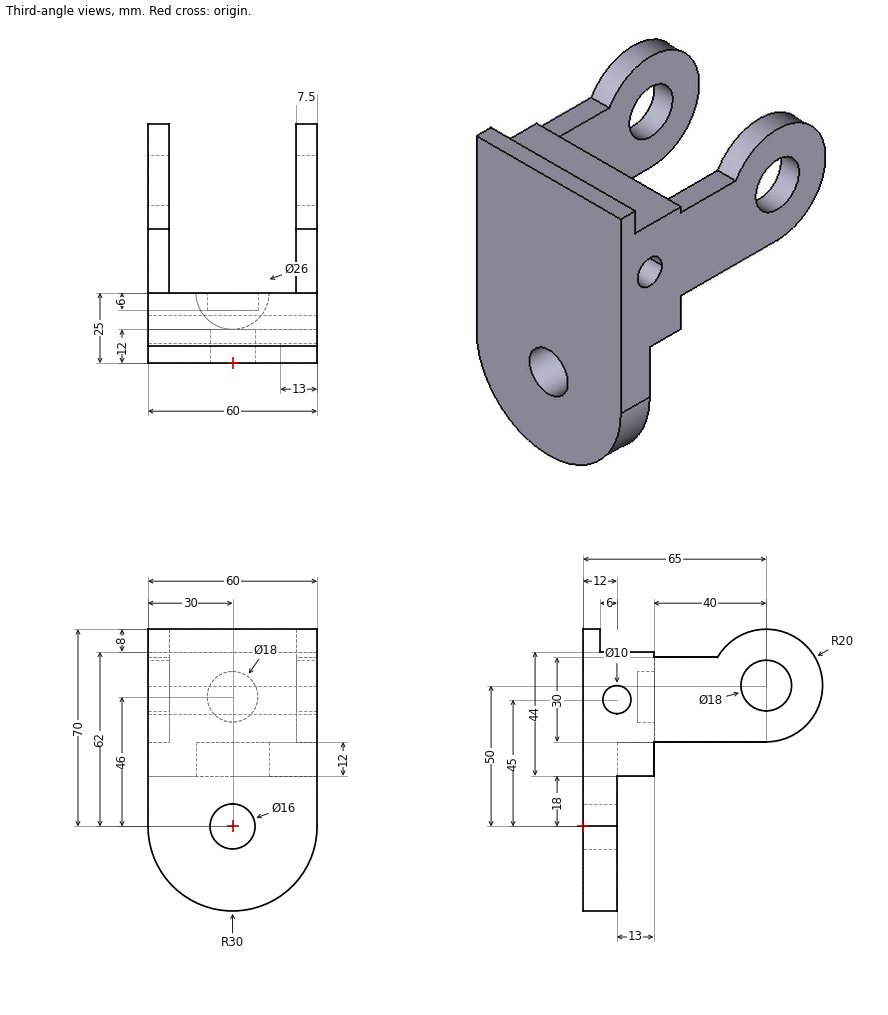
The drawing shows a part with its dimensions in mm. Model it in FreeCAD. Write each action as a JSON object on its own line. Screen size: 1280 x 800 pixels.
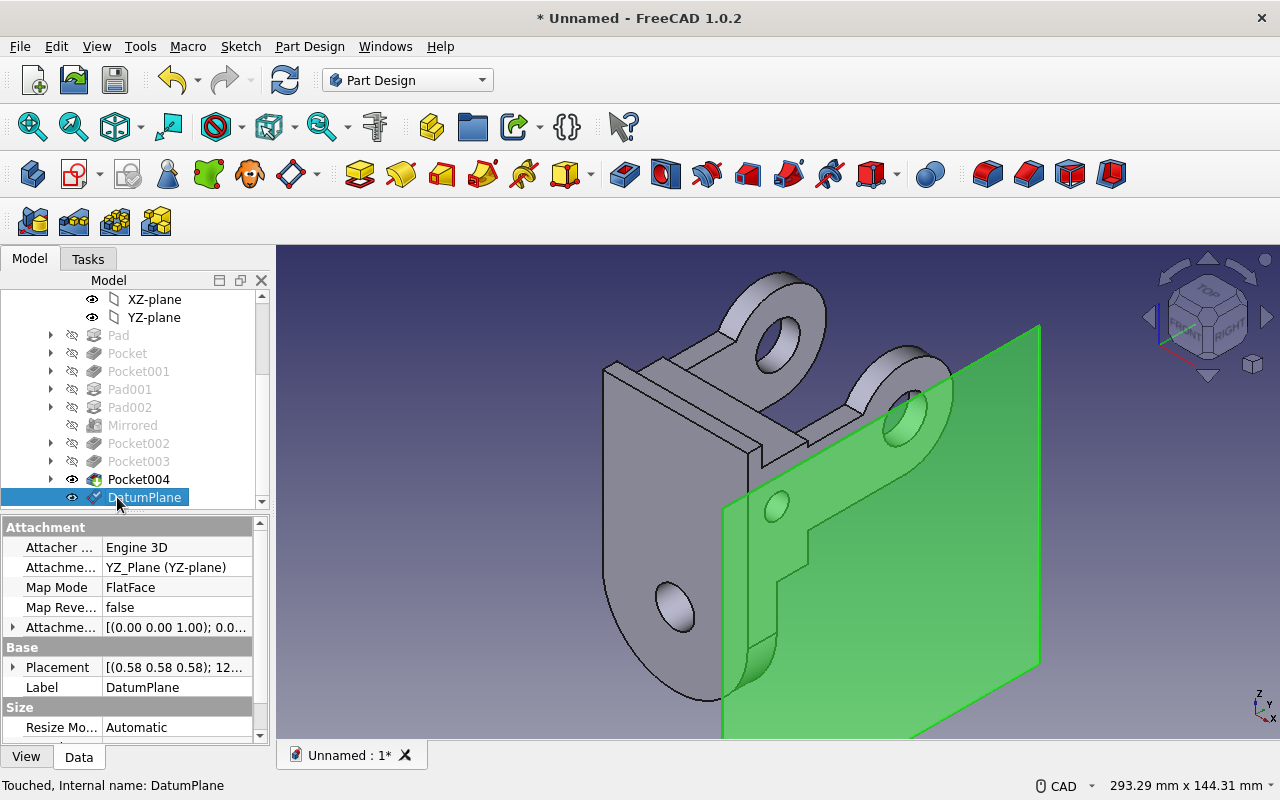
{"action": "left_click", "coordinate": [74, 174]}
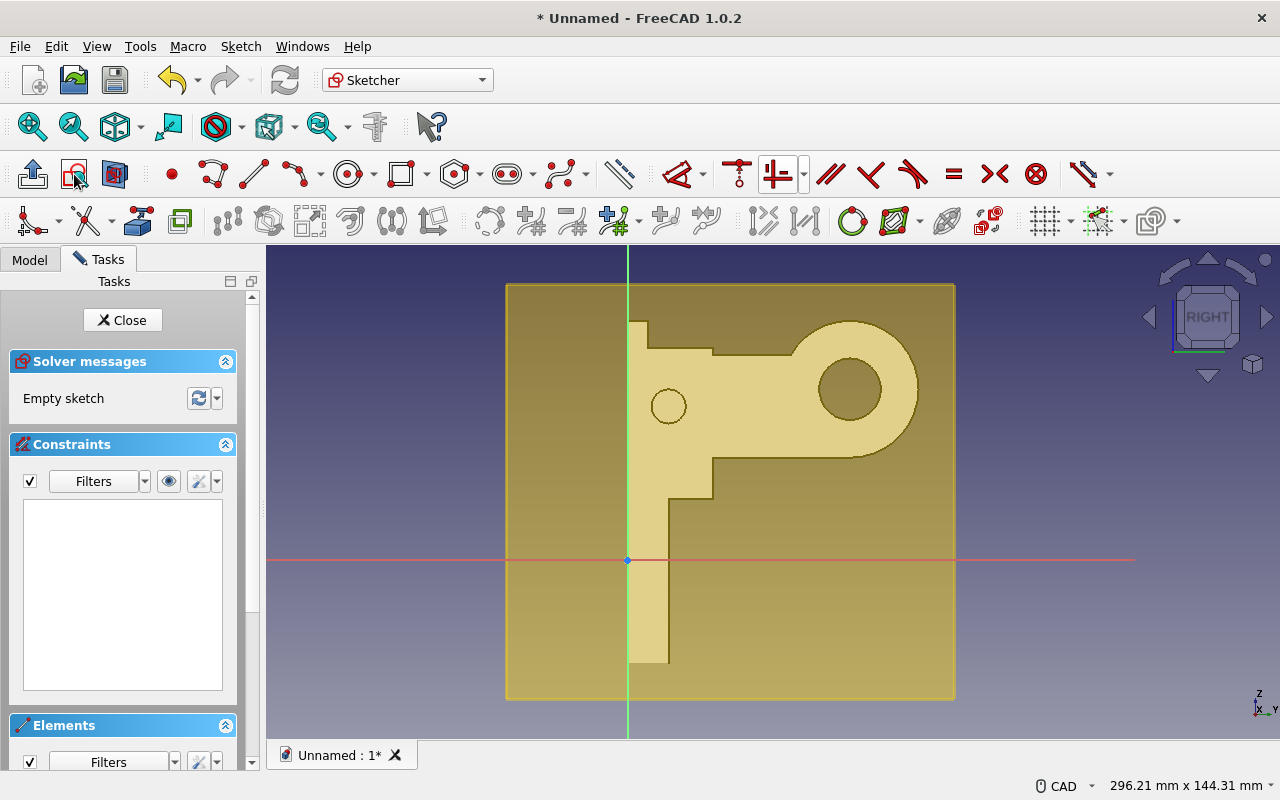
{"action": "scroll", "coordinate": [664, 396], "scroll_direction": "up", "scroll_amount": 11}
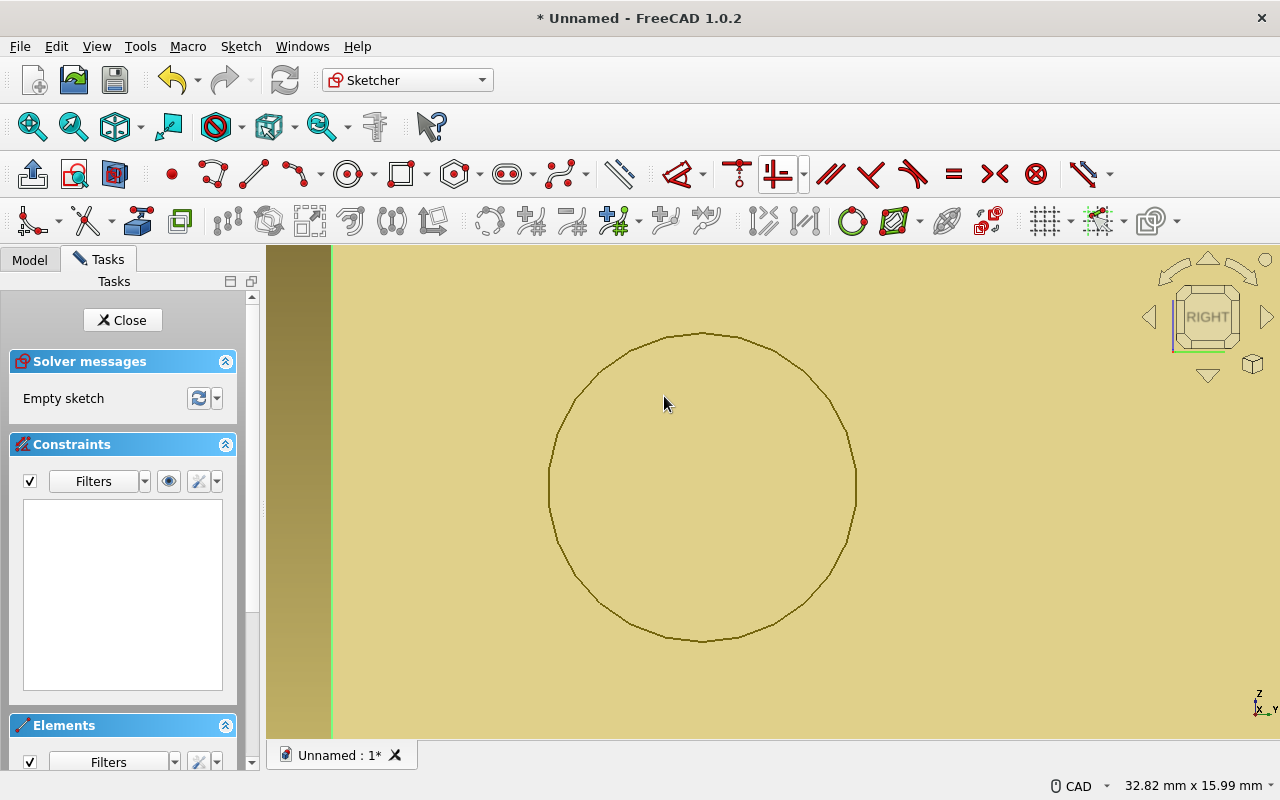
{"action": "left_click", "coordinate": [348, 174]}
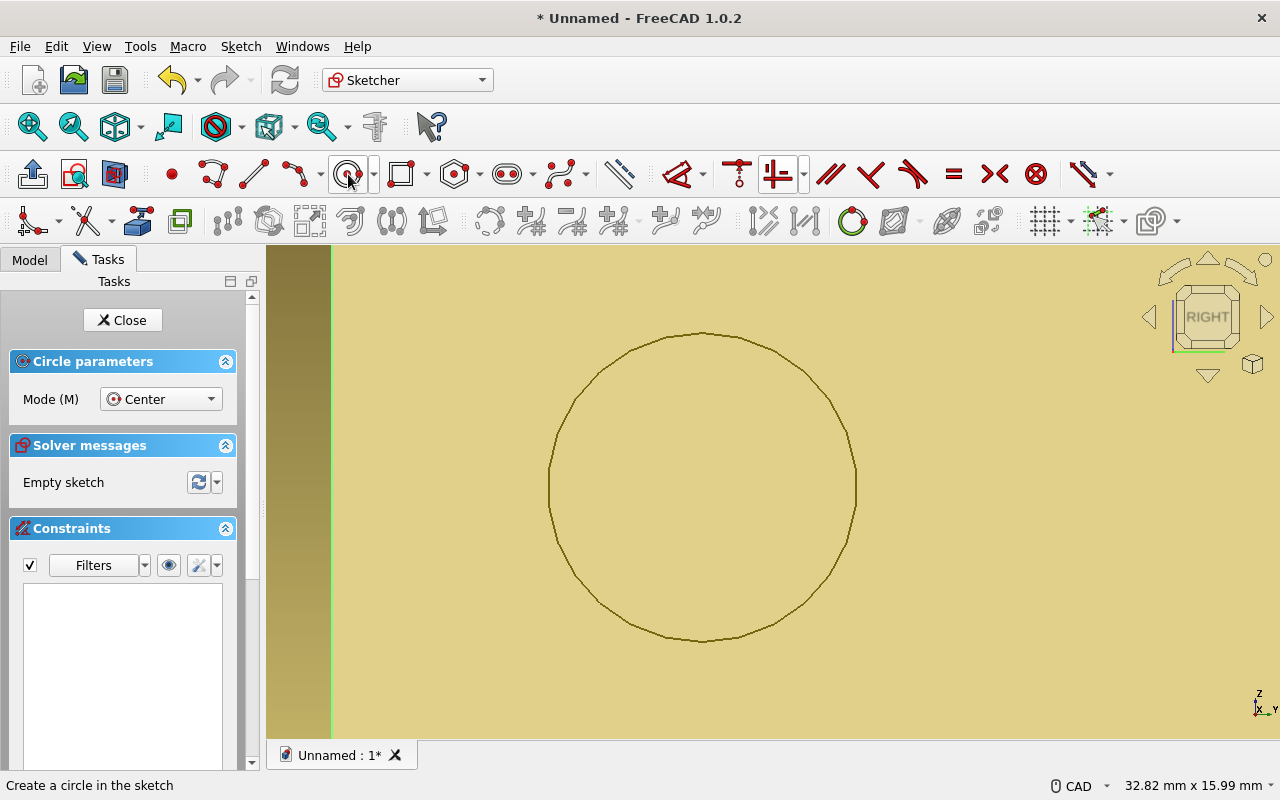
{"action": "left_click", "coordinate": [702, 488]}
{"action": "left_click", "coordinate": [812, 378]}
{"action": "key", "text": "Escape"}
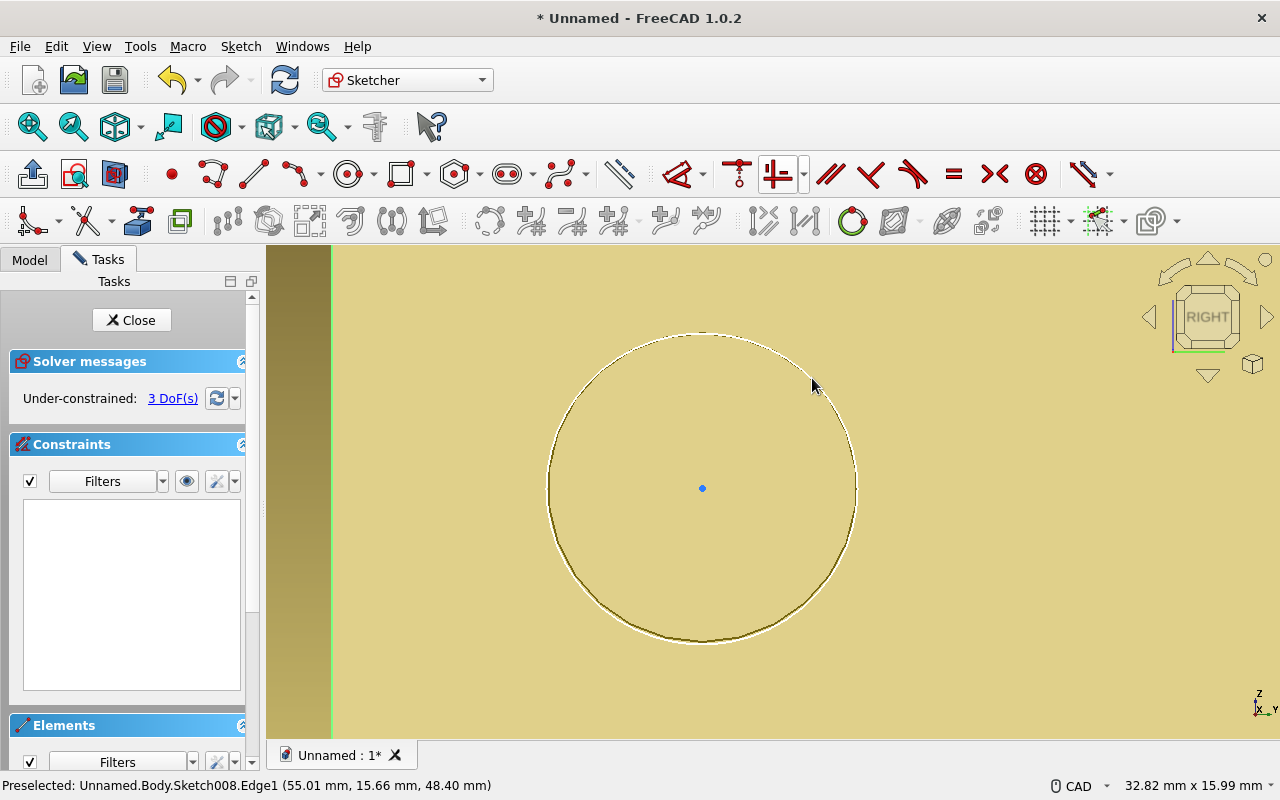
{"action": "key", "text": "d"}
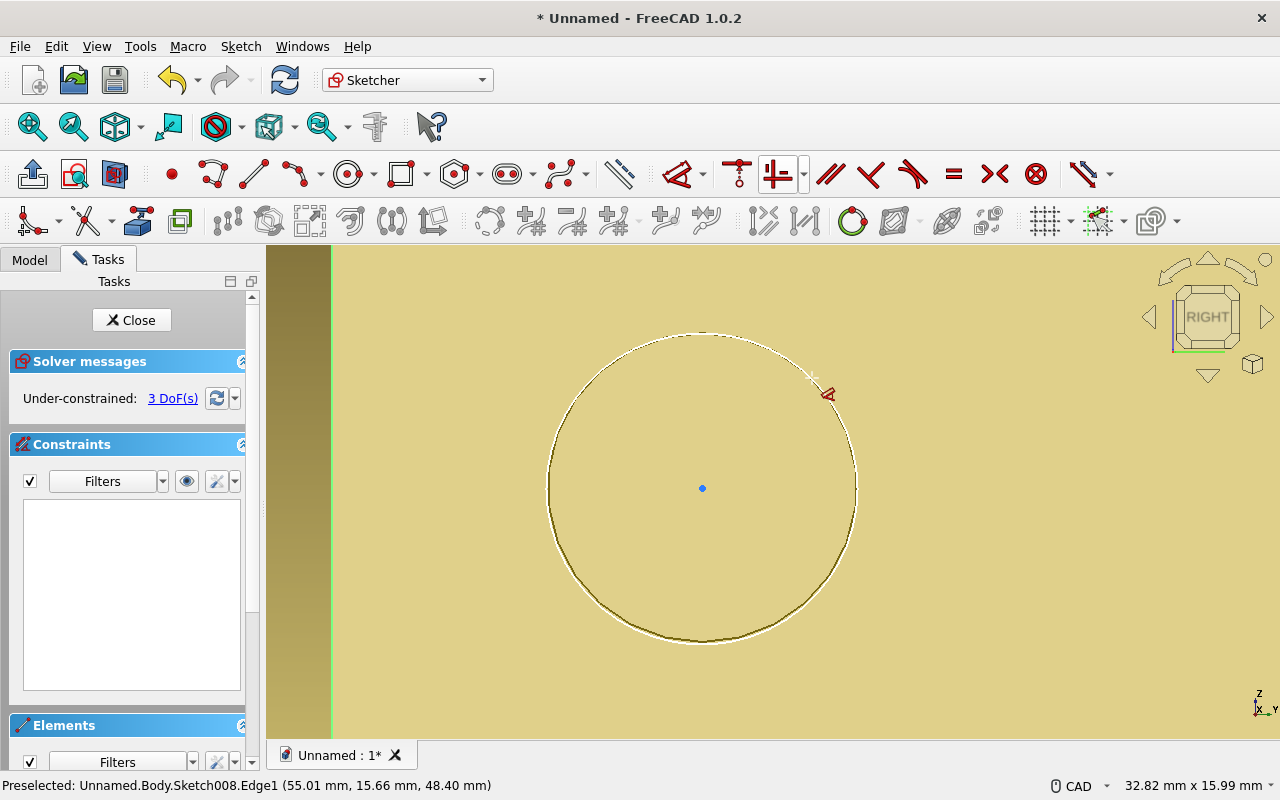
{"action": "left_click", "coordinate": [812, 379]}
{"action": "left_click", "coordinate": [835, 356]}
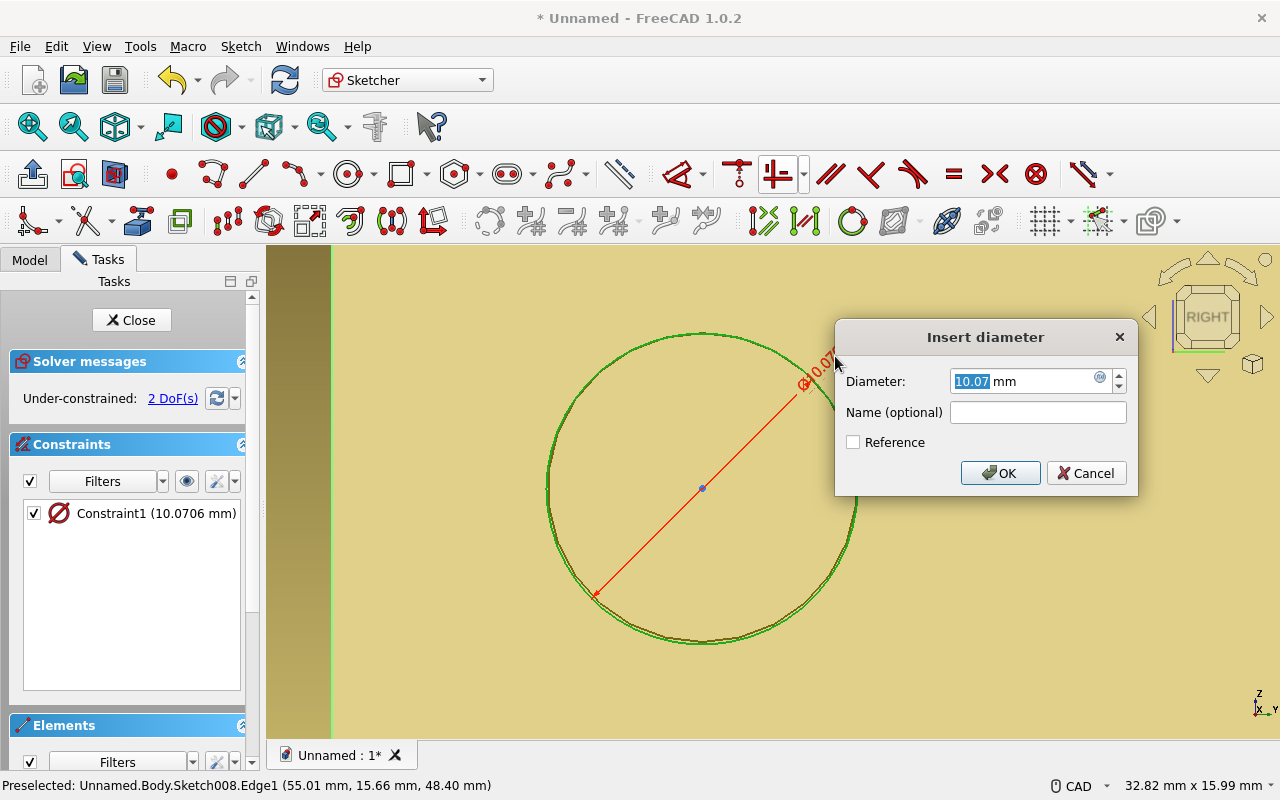
{"action": "type", "text": "10"}
{"action": "key", "text": "Return"}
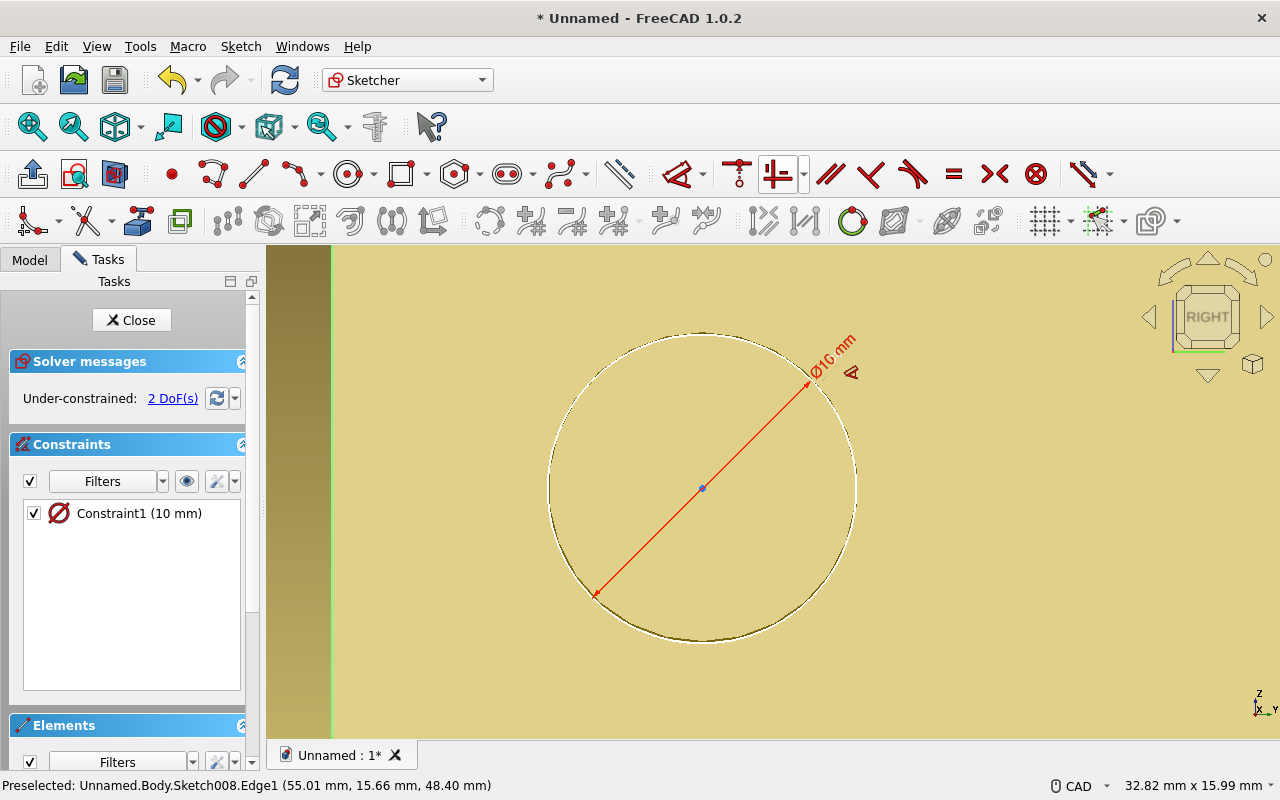
{"action": "left_click", "coordinate": [702, 489]}
{"action": "left_click", "coordinate": [517, 455]}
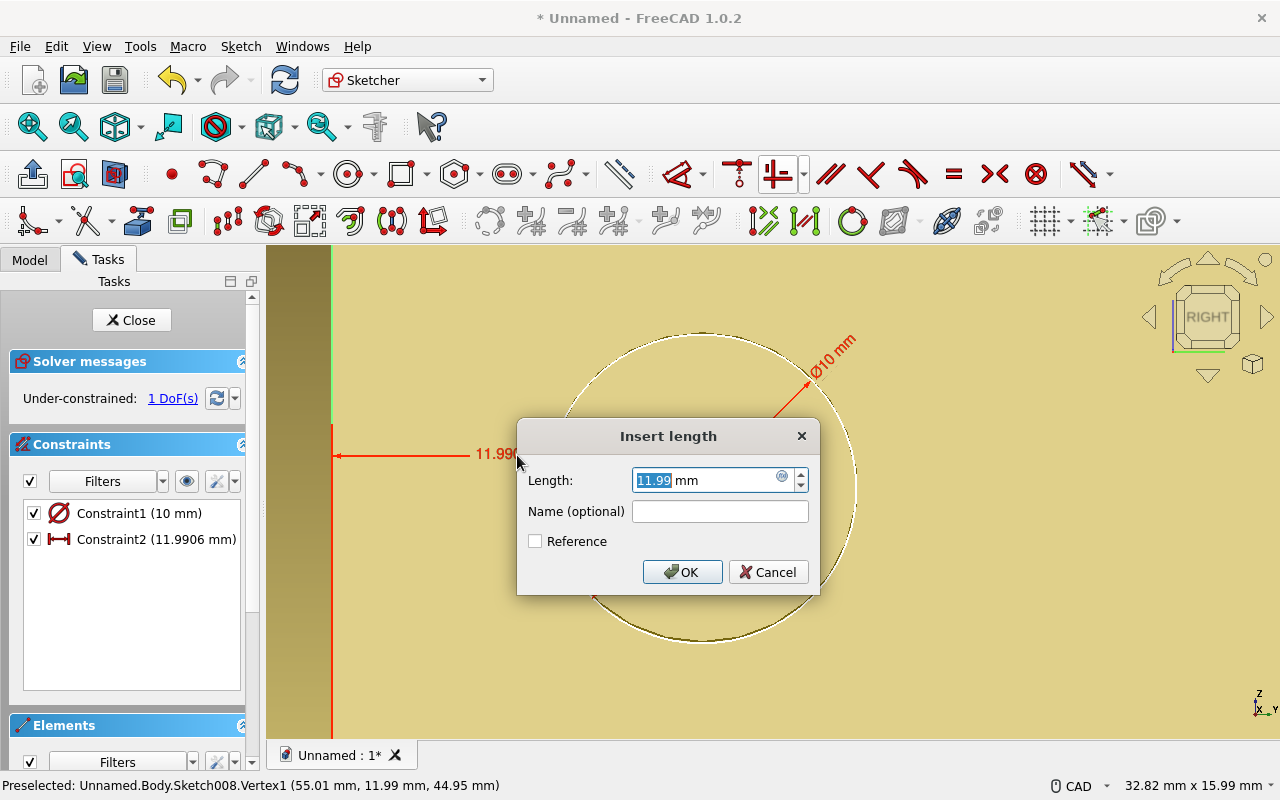
{"action": "type", "text": "12"}
{"action": "key", "text": "Return"}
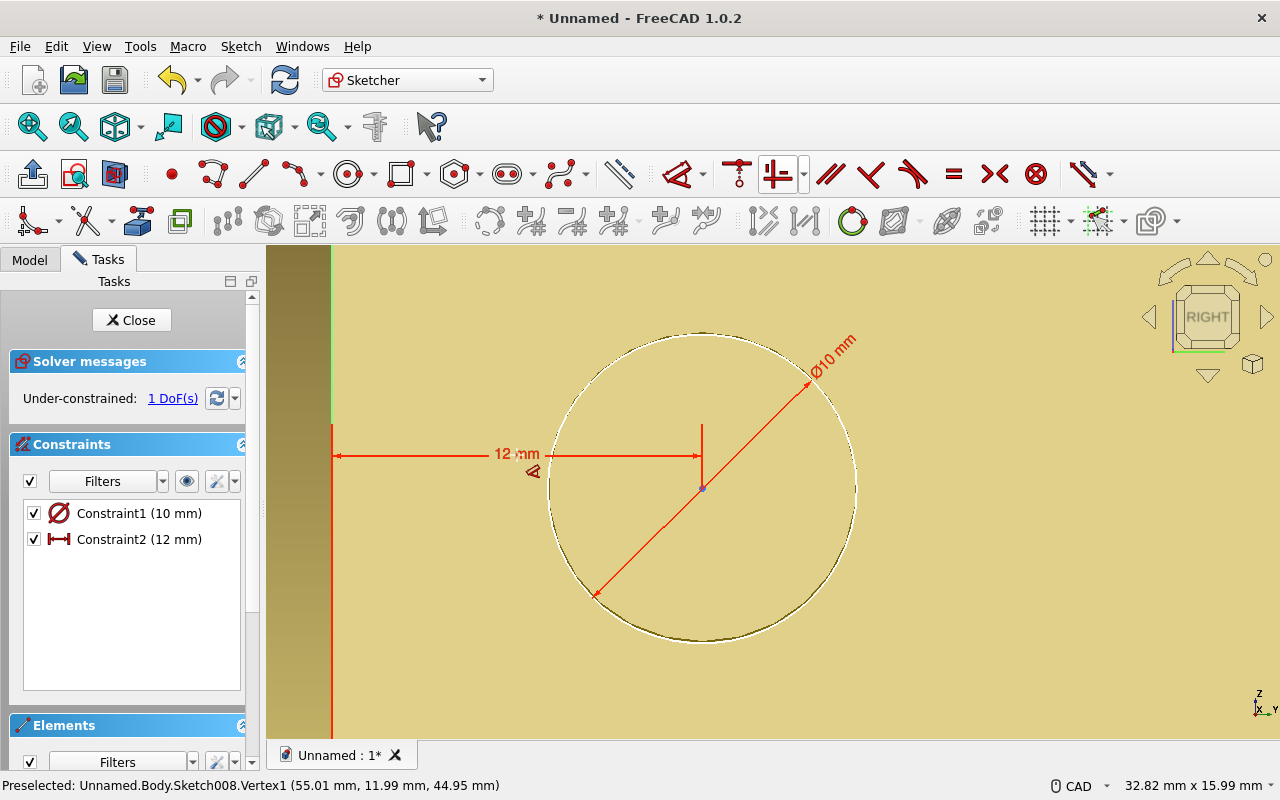
{"action": "left_click", "coordinate": [702, 489]}
{"action": "left_click", "coordinate": [298, 600]}